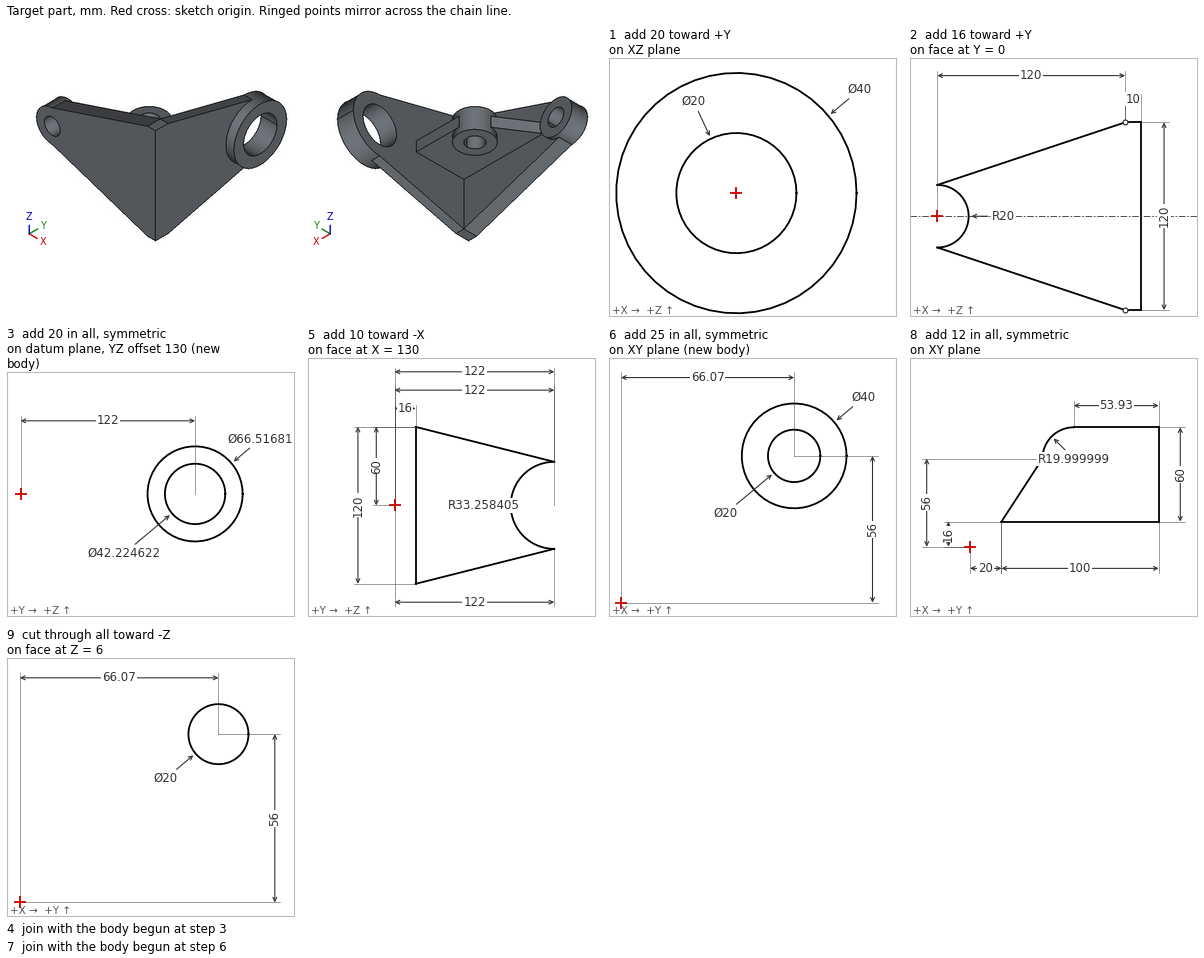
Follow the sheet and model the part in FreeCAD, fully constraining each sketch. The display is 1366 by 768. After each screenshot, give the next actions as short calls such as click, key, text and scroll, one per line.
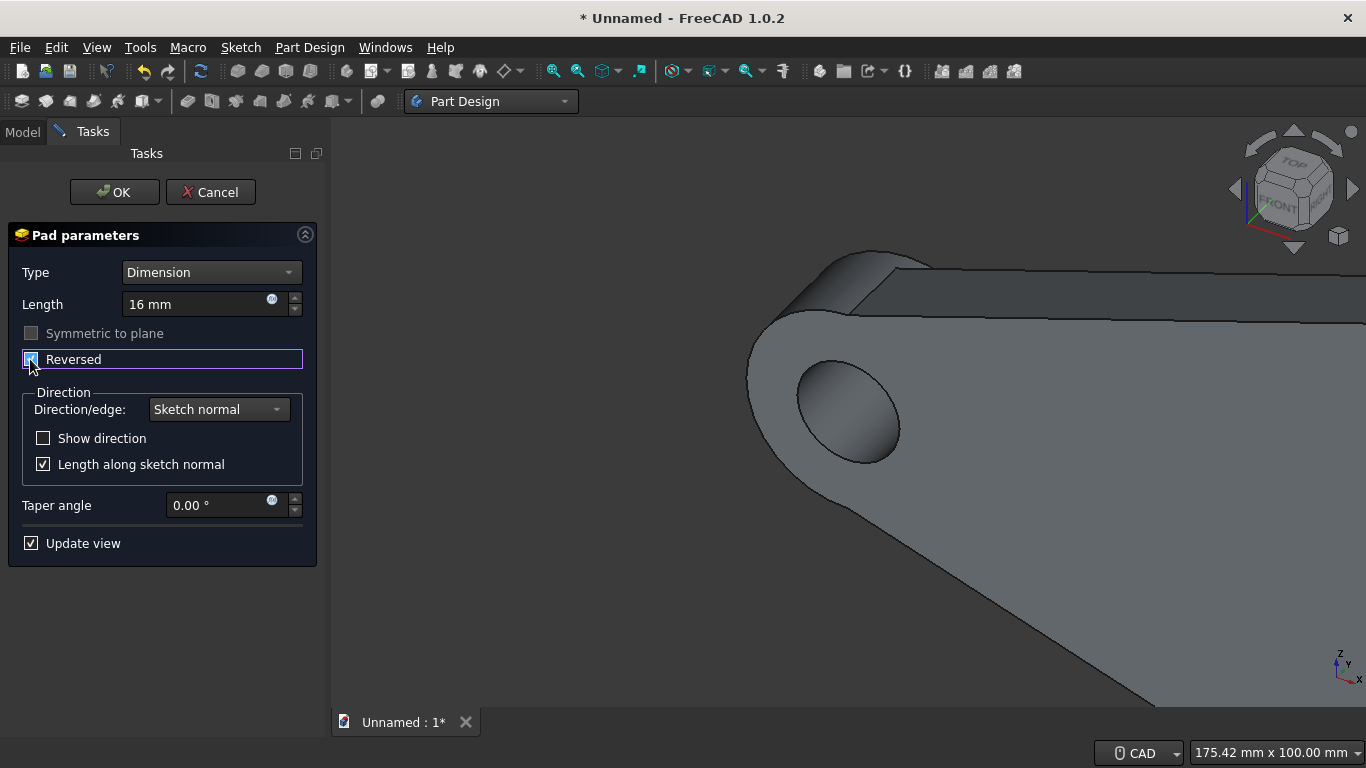
click(115, 192)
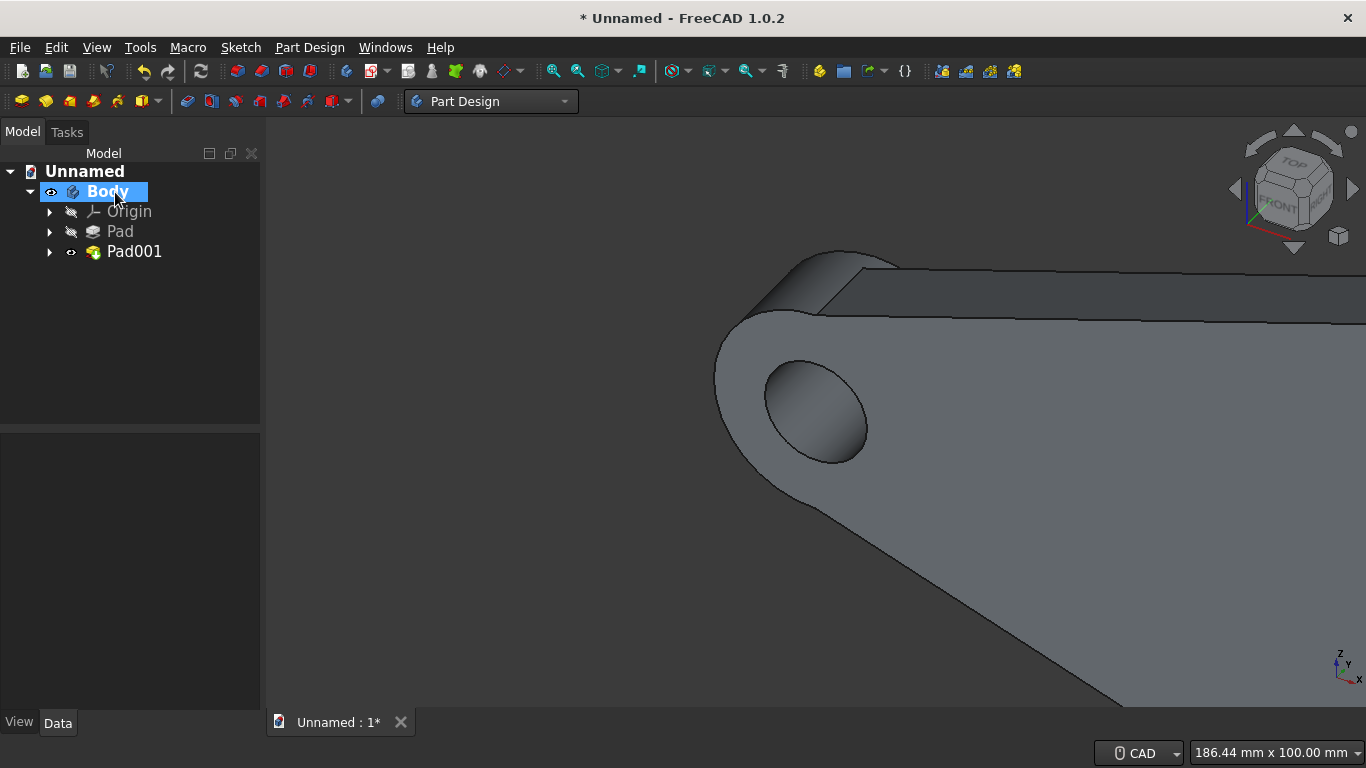
click(554, 72)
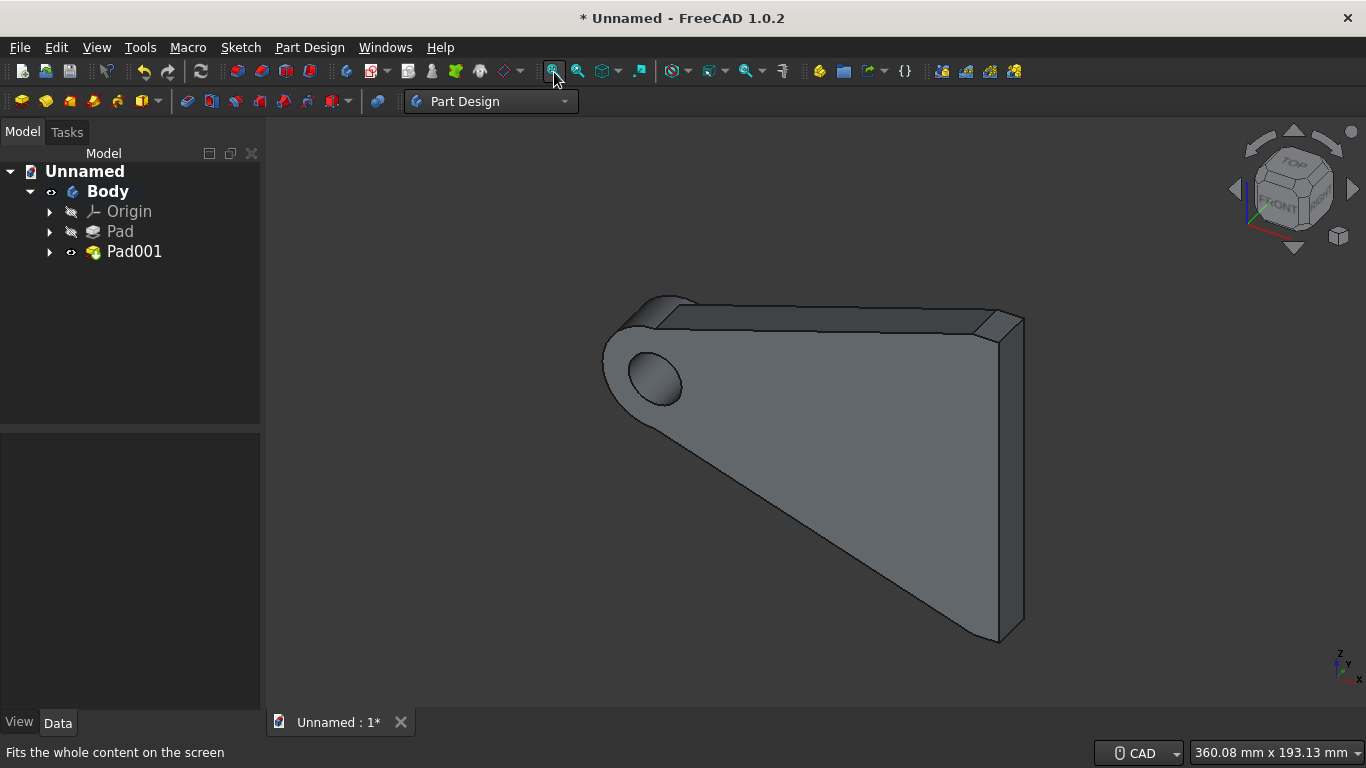
click(348, 72)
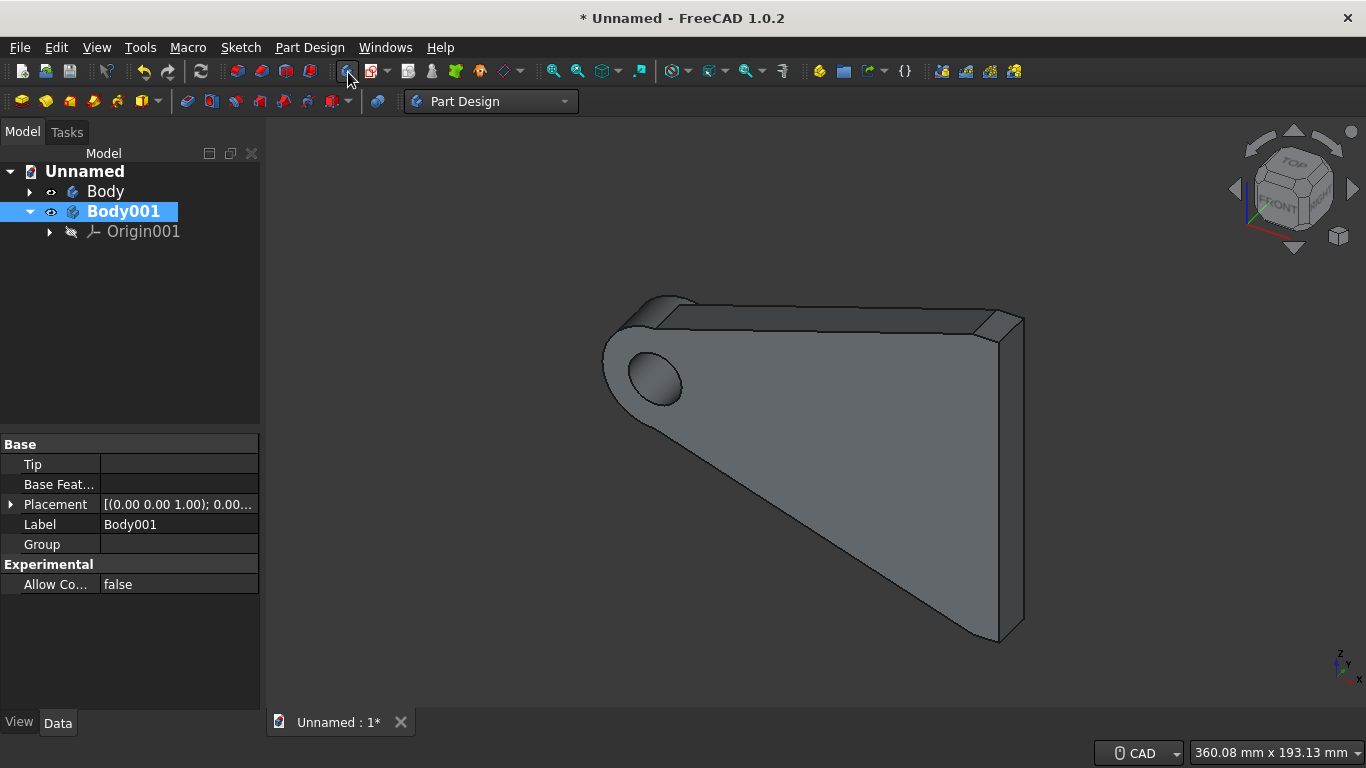
click(50, 232)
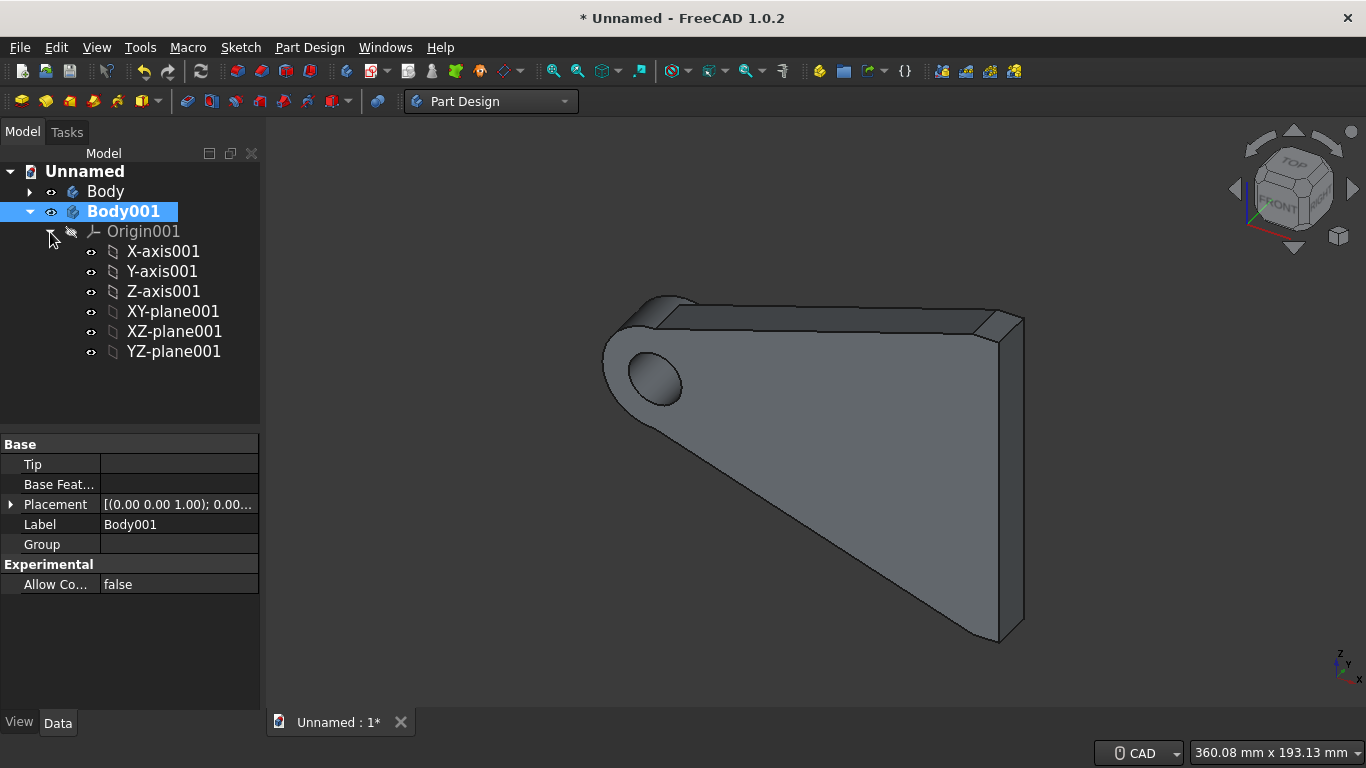
click(136, 352)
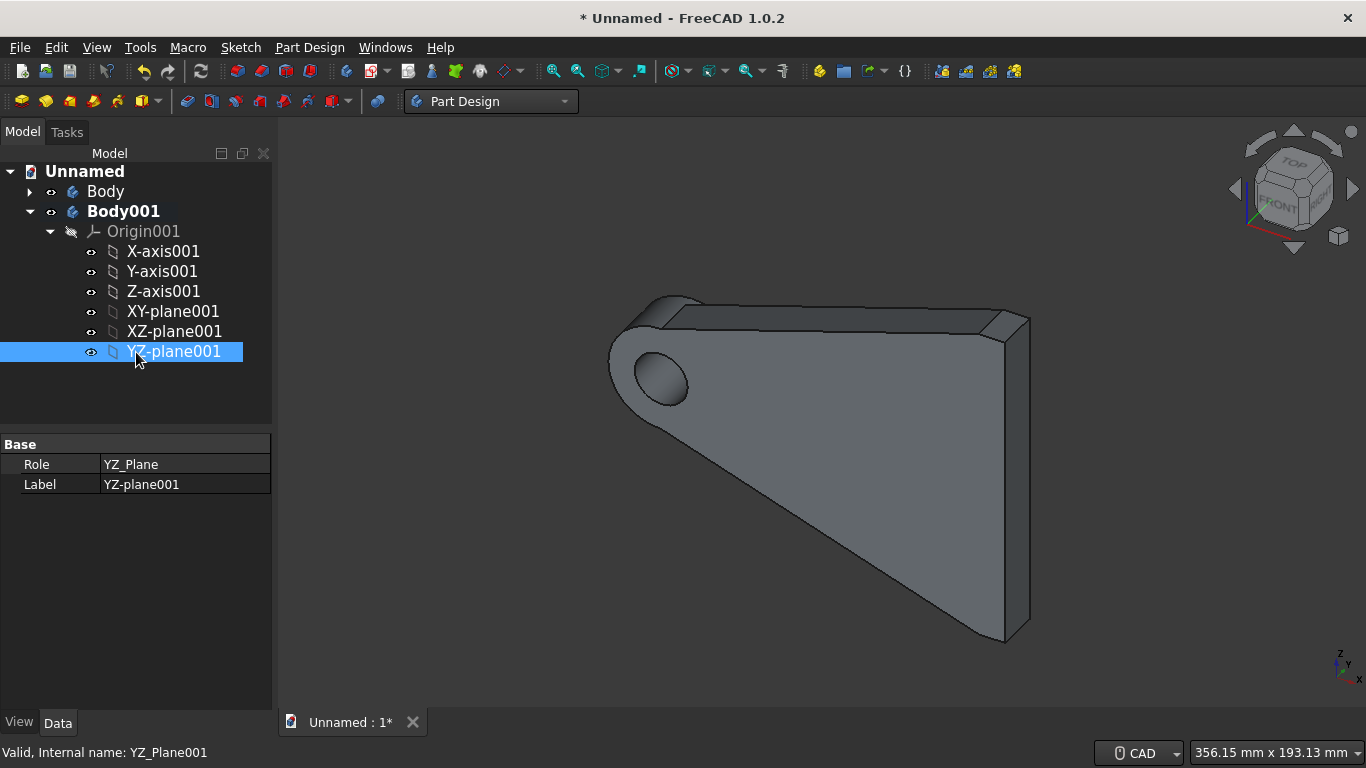
click(504, 72)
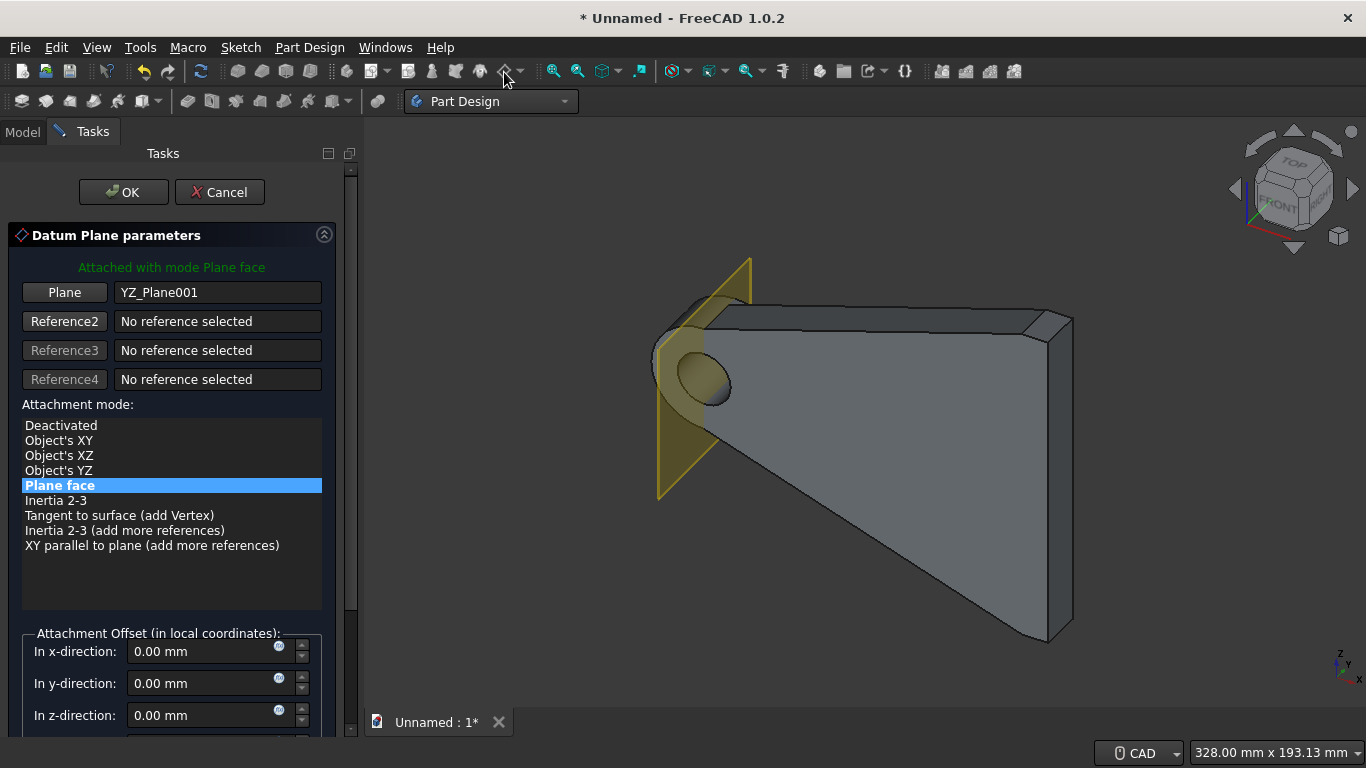
triple_click(210, 715)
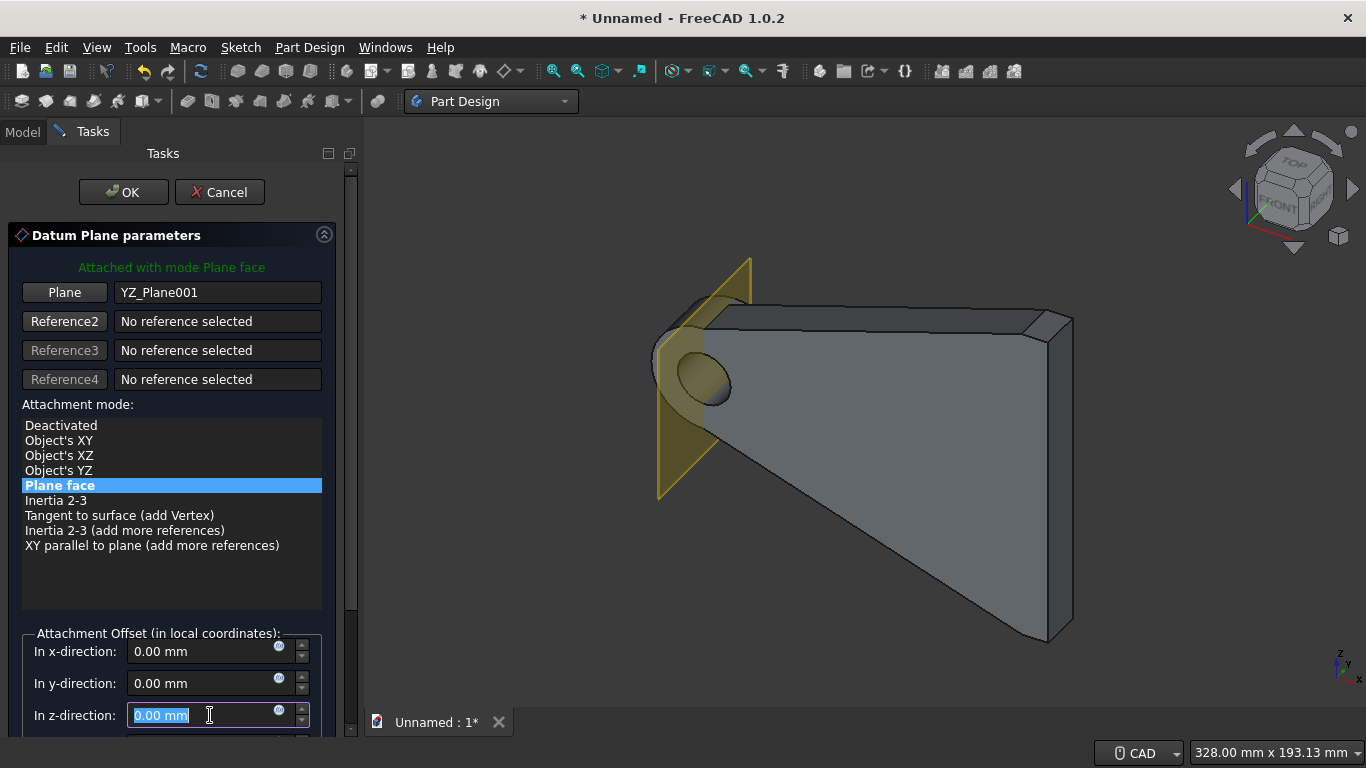
text(130)
key(Tab)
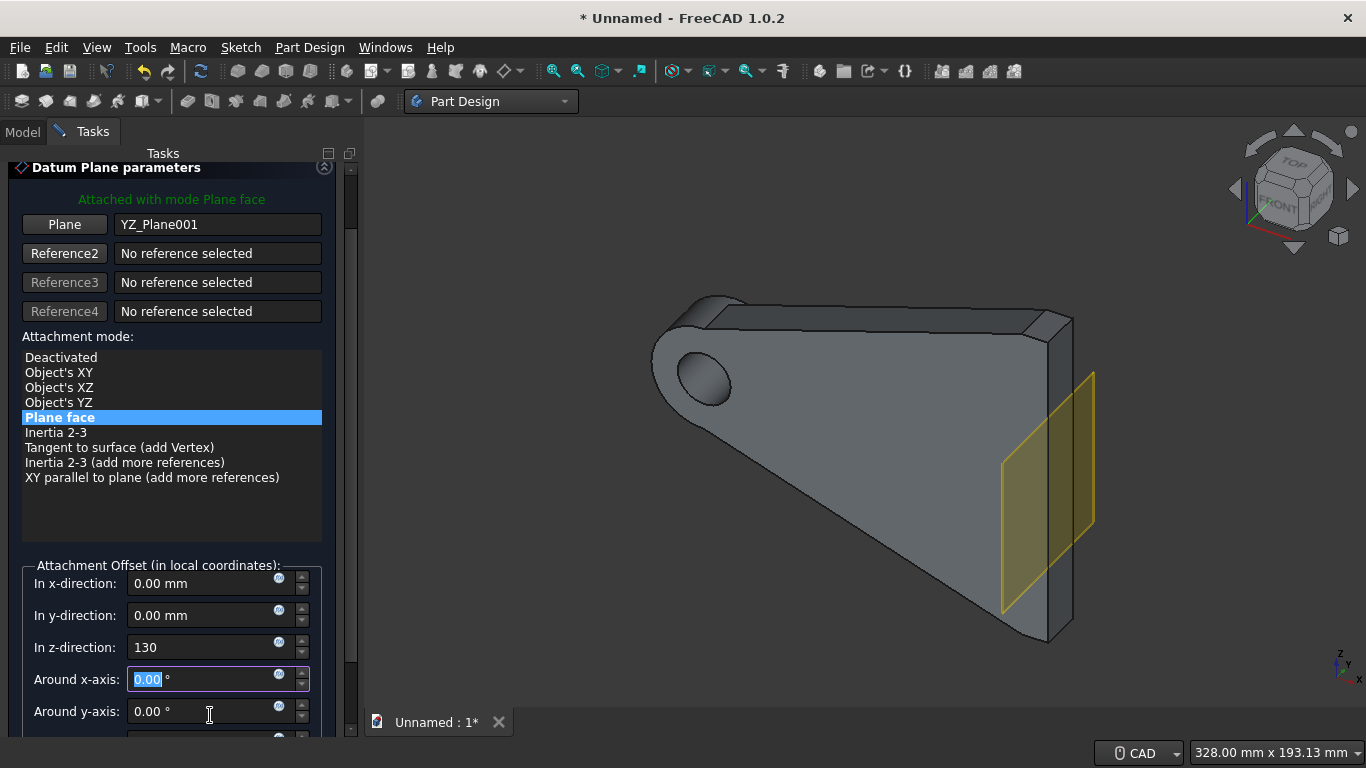
scroll(351, 450, up, 2)